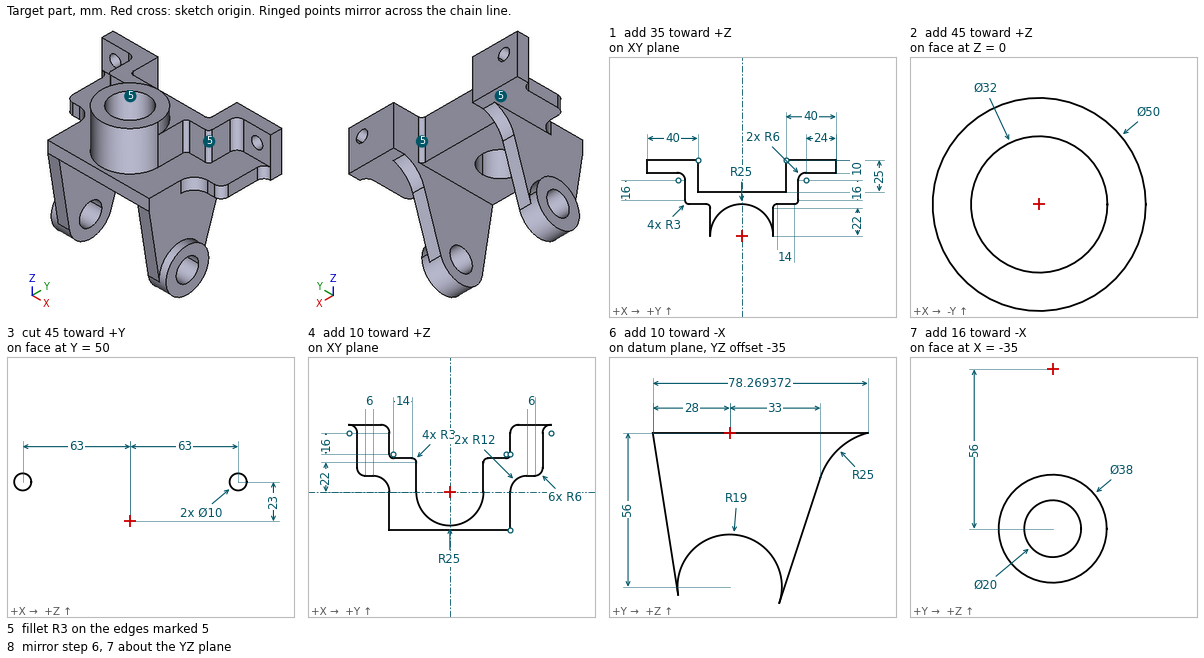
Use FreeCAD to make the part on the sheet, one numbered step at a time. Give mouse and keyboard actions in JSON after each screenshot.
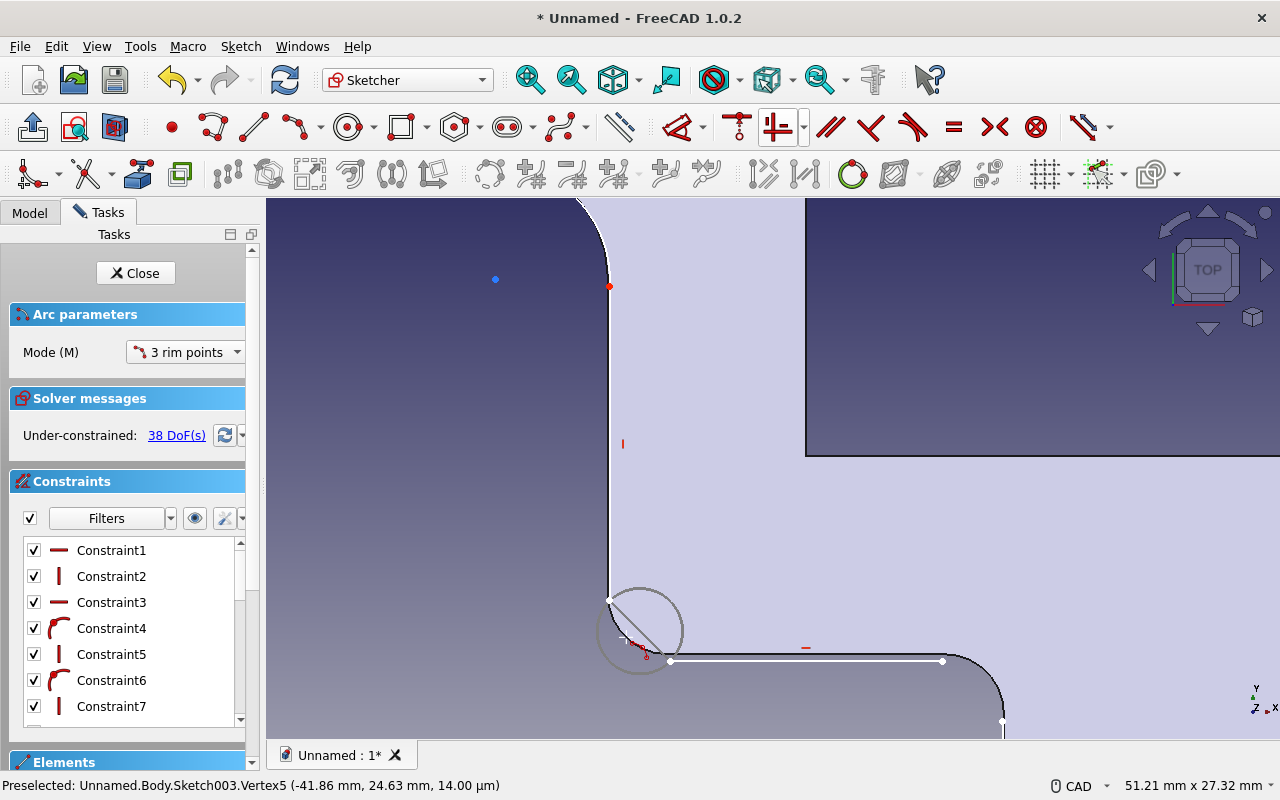
{"action": "left_click", "coordinate": [625, 637]}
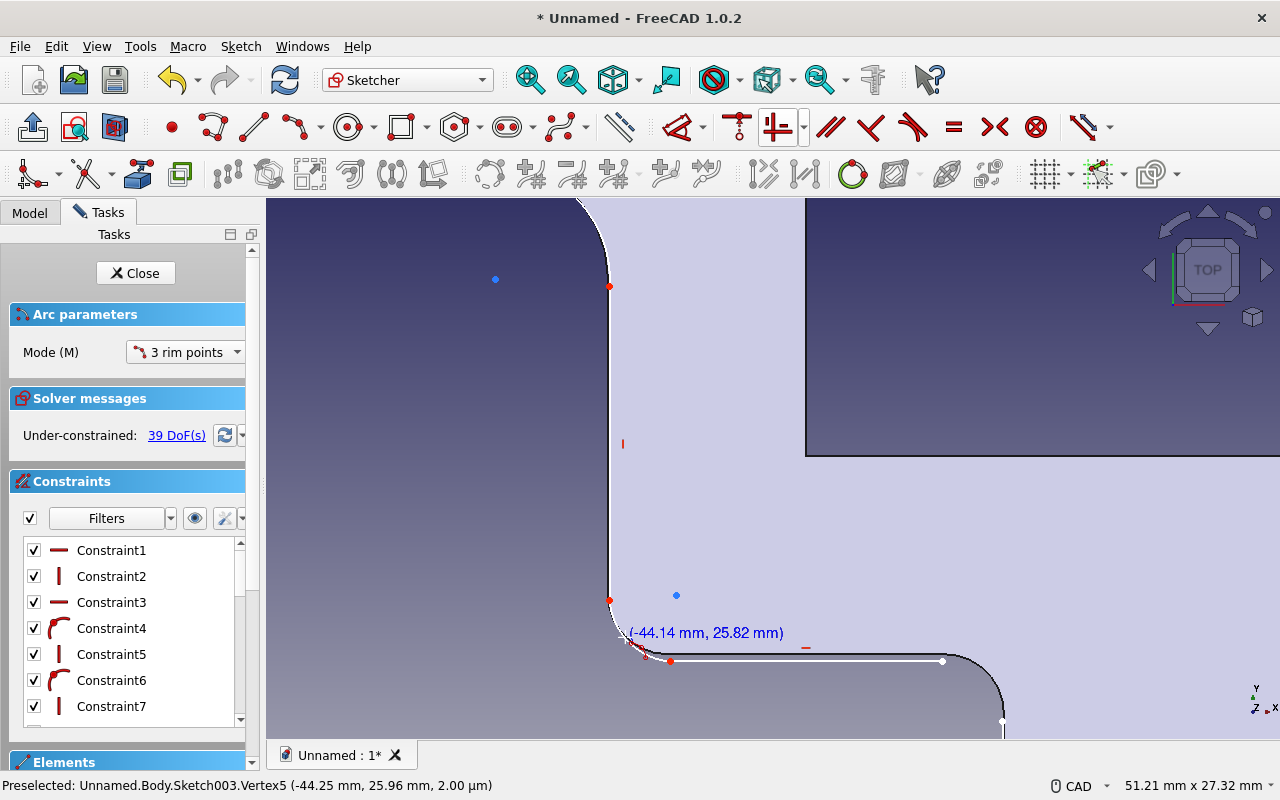
{"action": "scroll", "coordinate": [504, 351], "scroll_direction": "down", "scroll_amount": 8}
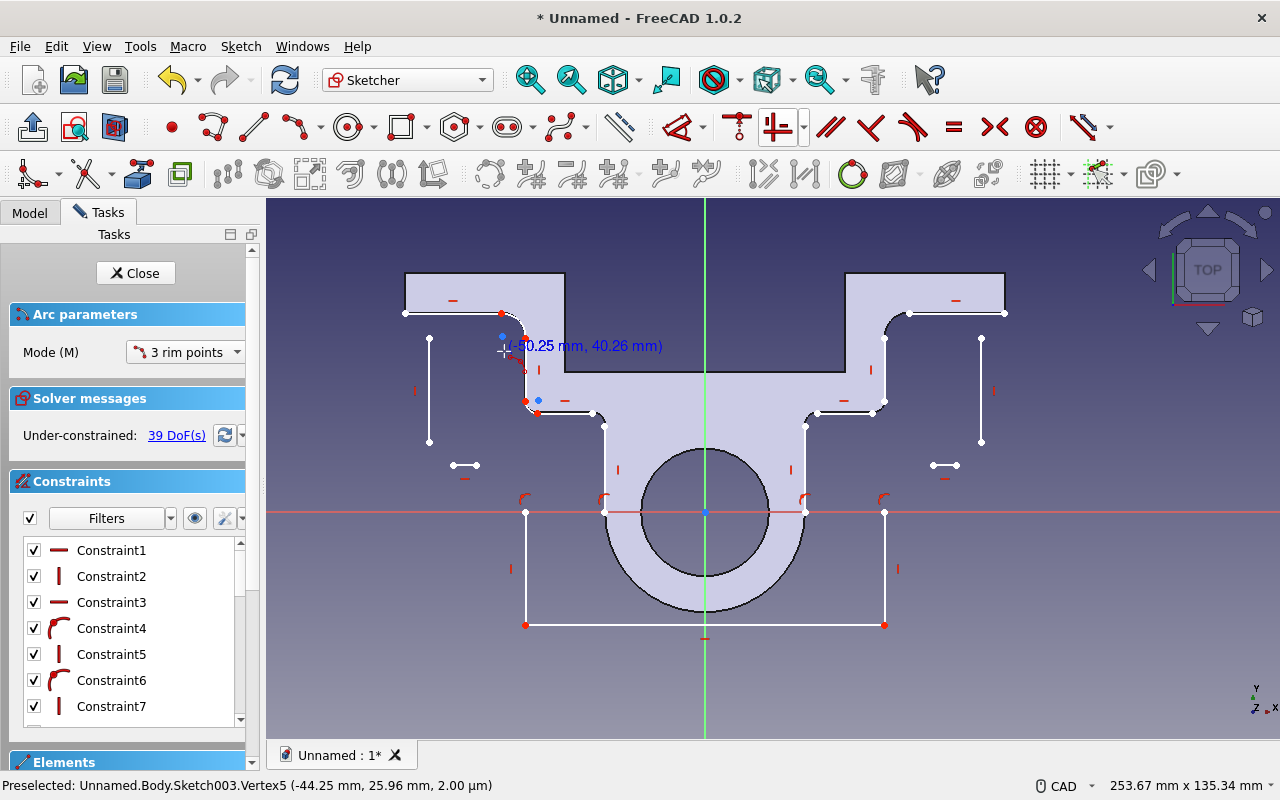
{"action": "left_click", "coordinate": [593, 414]}
{"action": "left_click", "coordinate": [605, 426]}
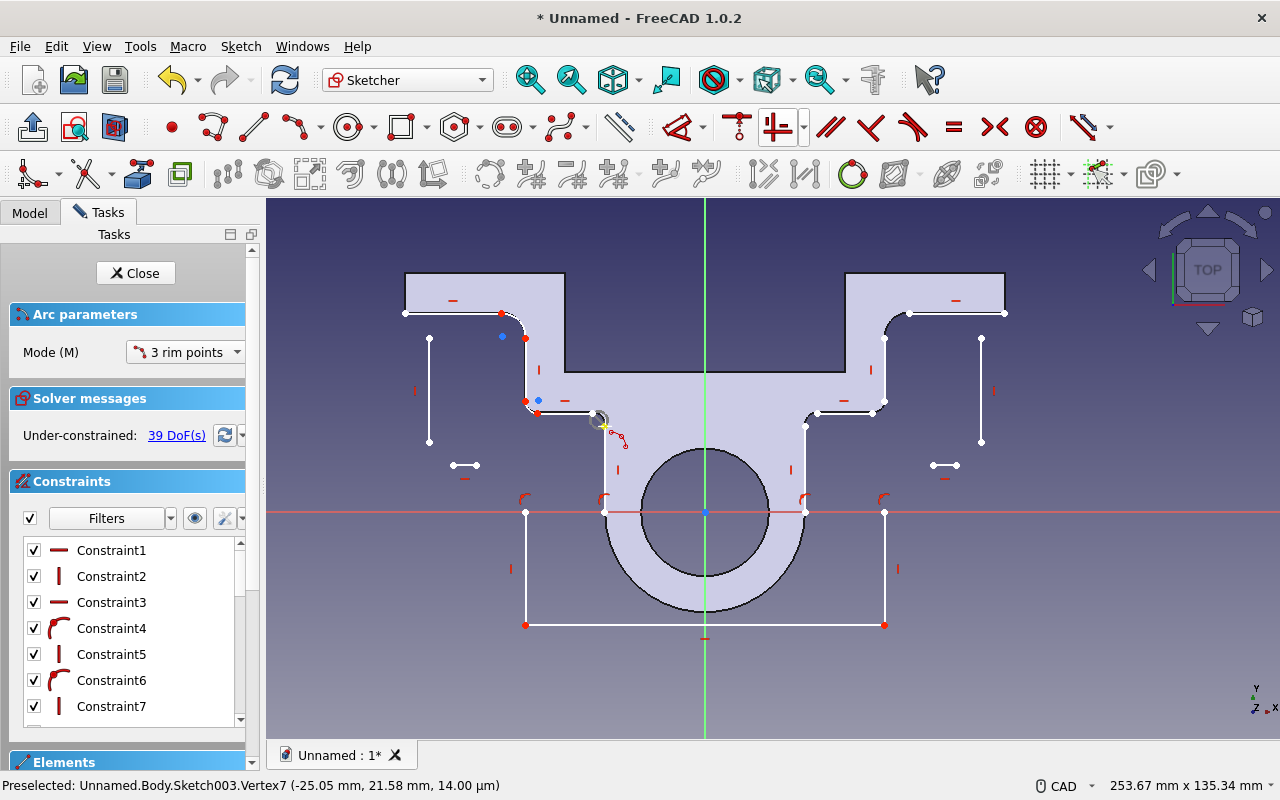
{"action": "scroll", "coordinate": [602, 416], "scroll_direction": "up", "scroll_amount": 8}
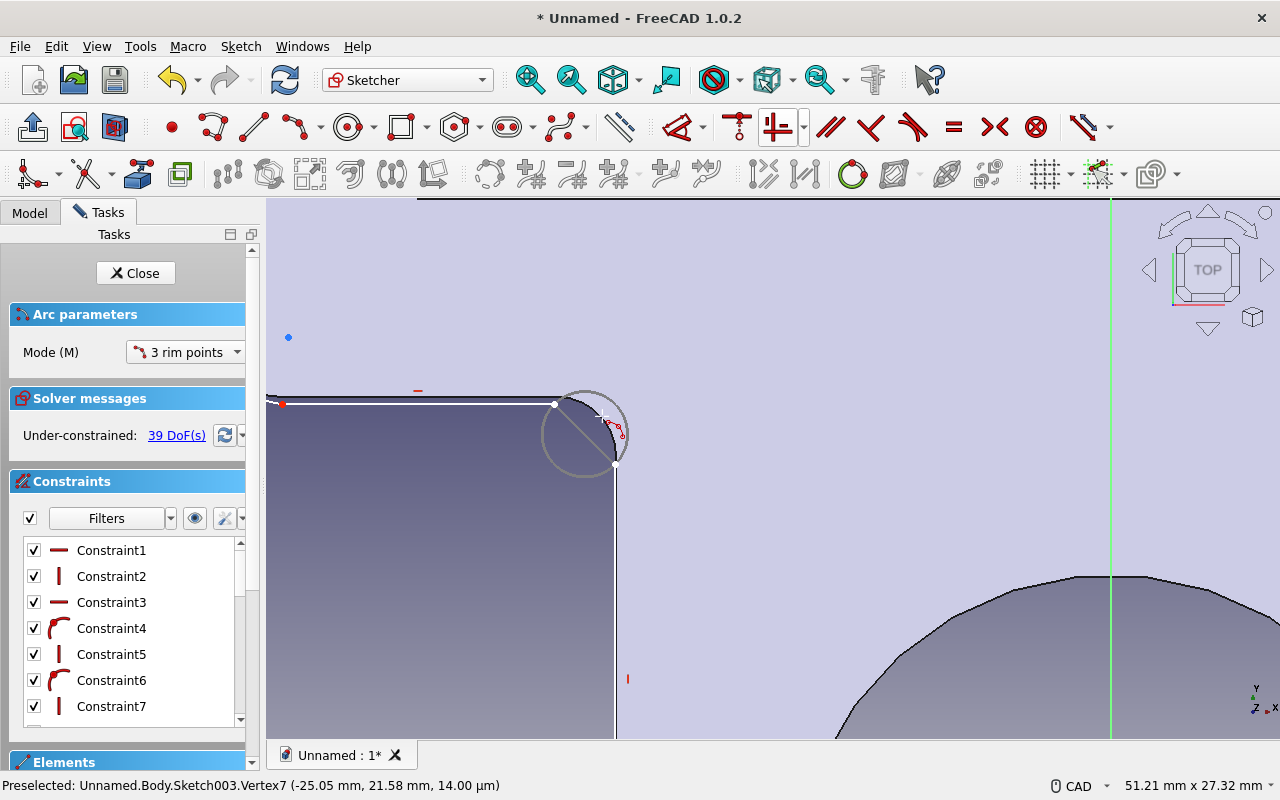
{"action": "left_click", "coordinate": [599, 414]}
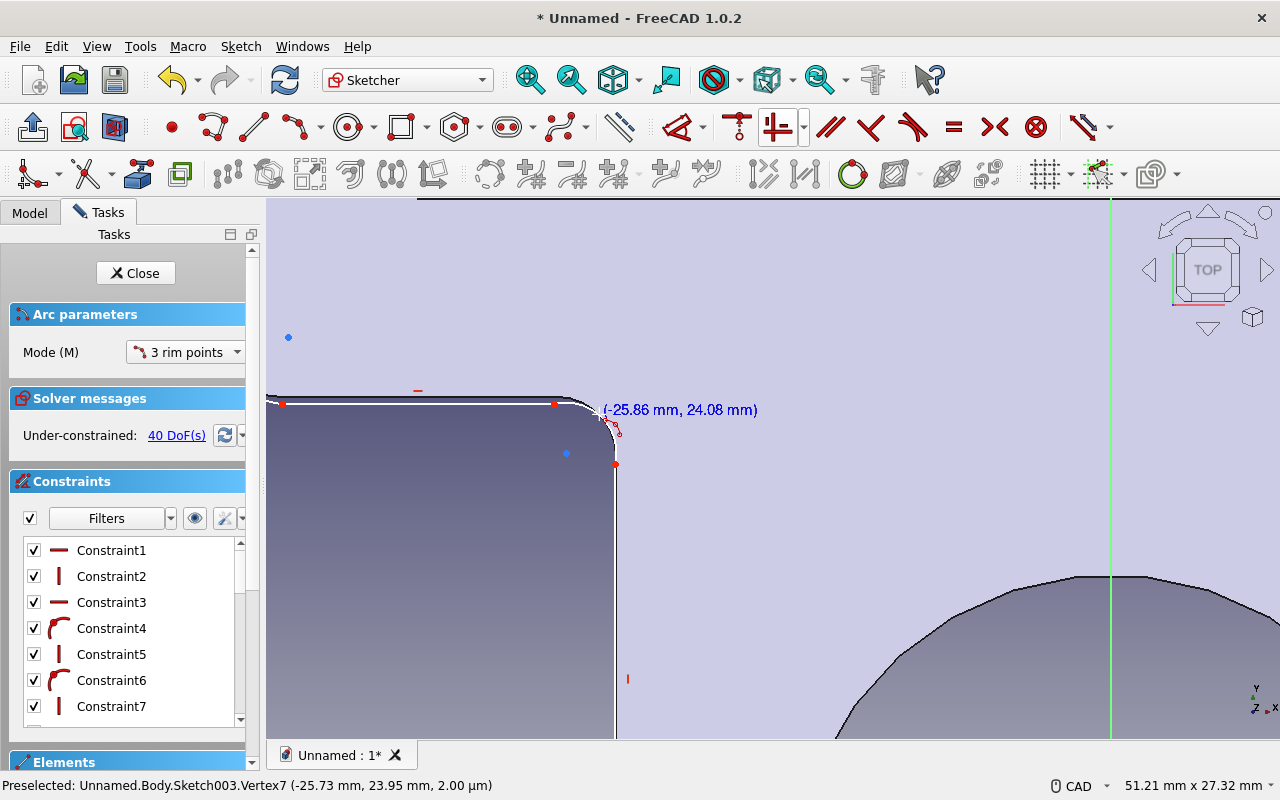
{"action": "scroll", "coordinate": [602, 417], "scroll_direction": "down", "scroll_amount": 8}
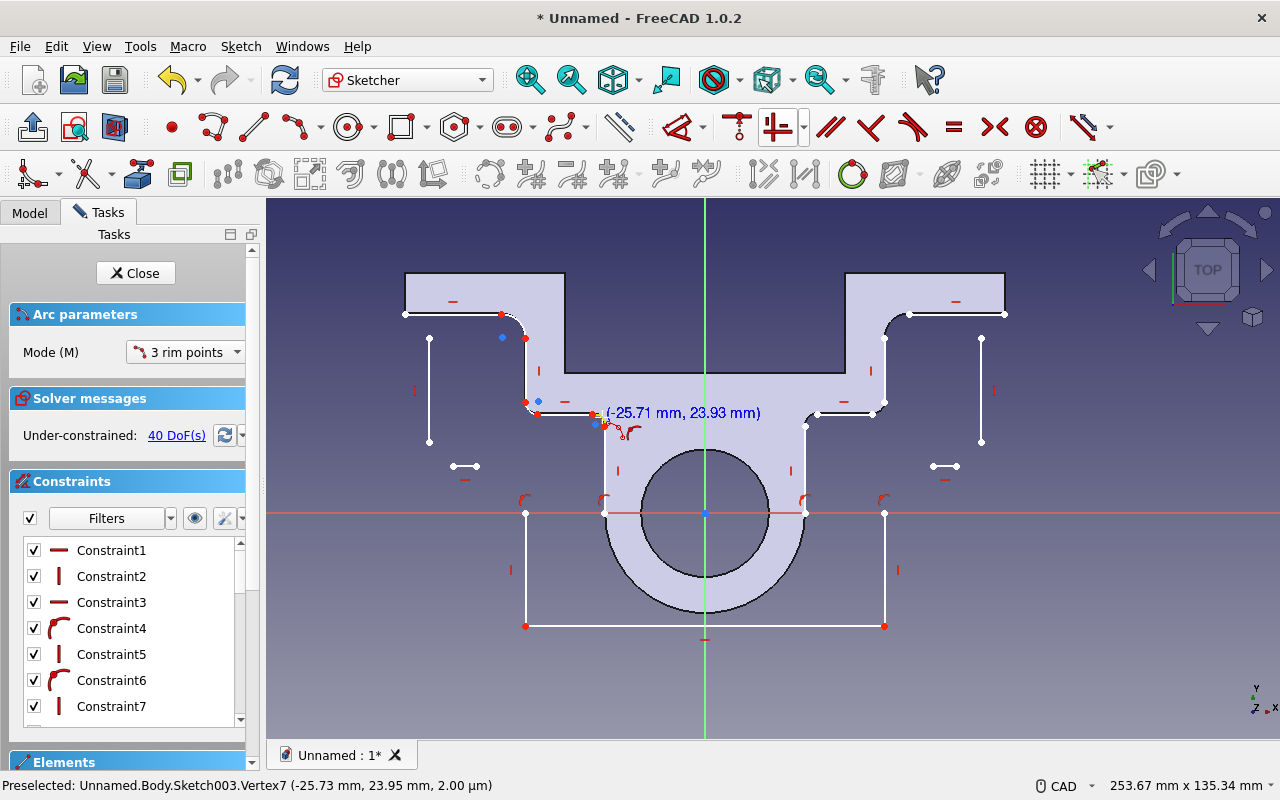
{"action": "left_click", "coordinate": [605, 513]}
{"action": "left_click", "coordinate": [805, 513]}
{"action": "left_click", "coordinate": [646, 594]}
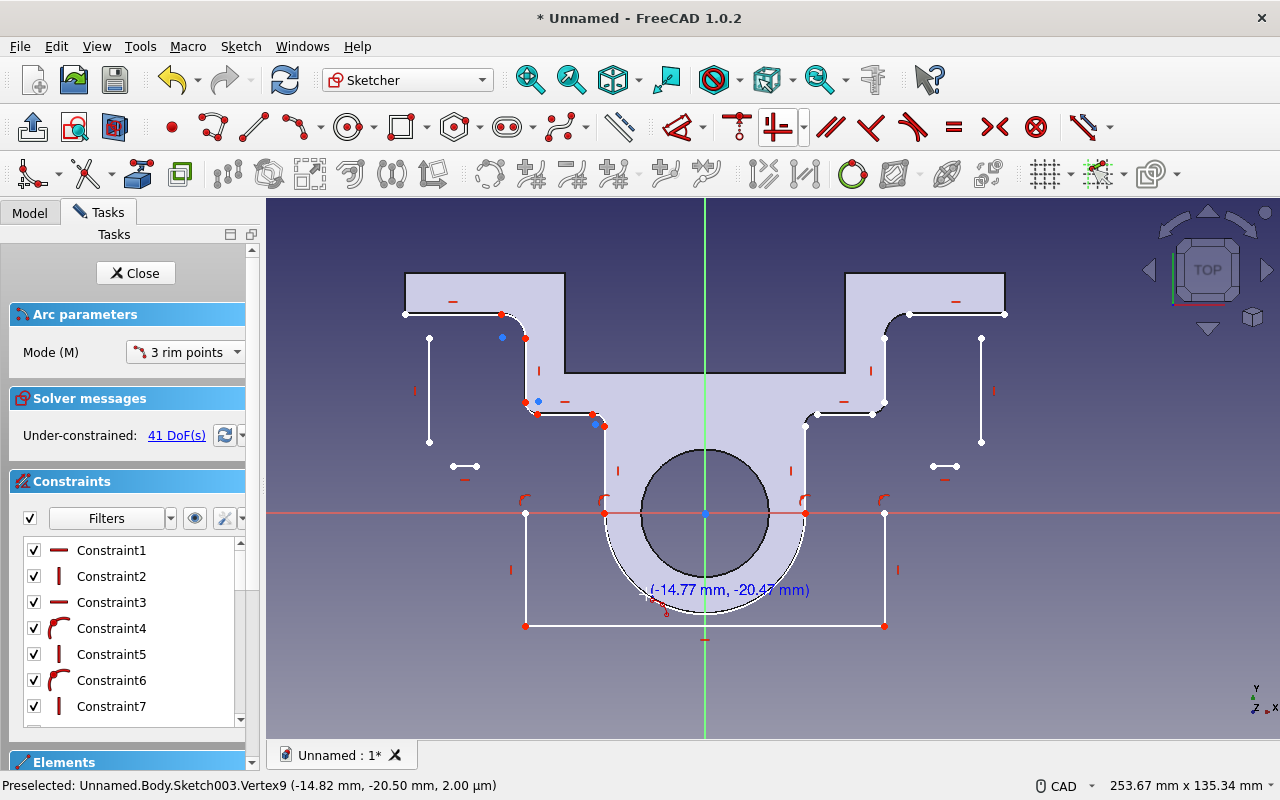
{"action": "left_click", "coordinate": [805, 427]}
{"action": "left_click", "coordinate": [817, 415]}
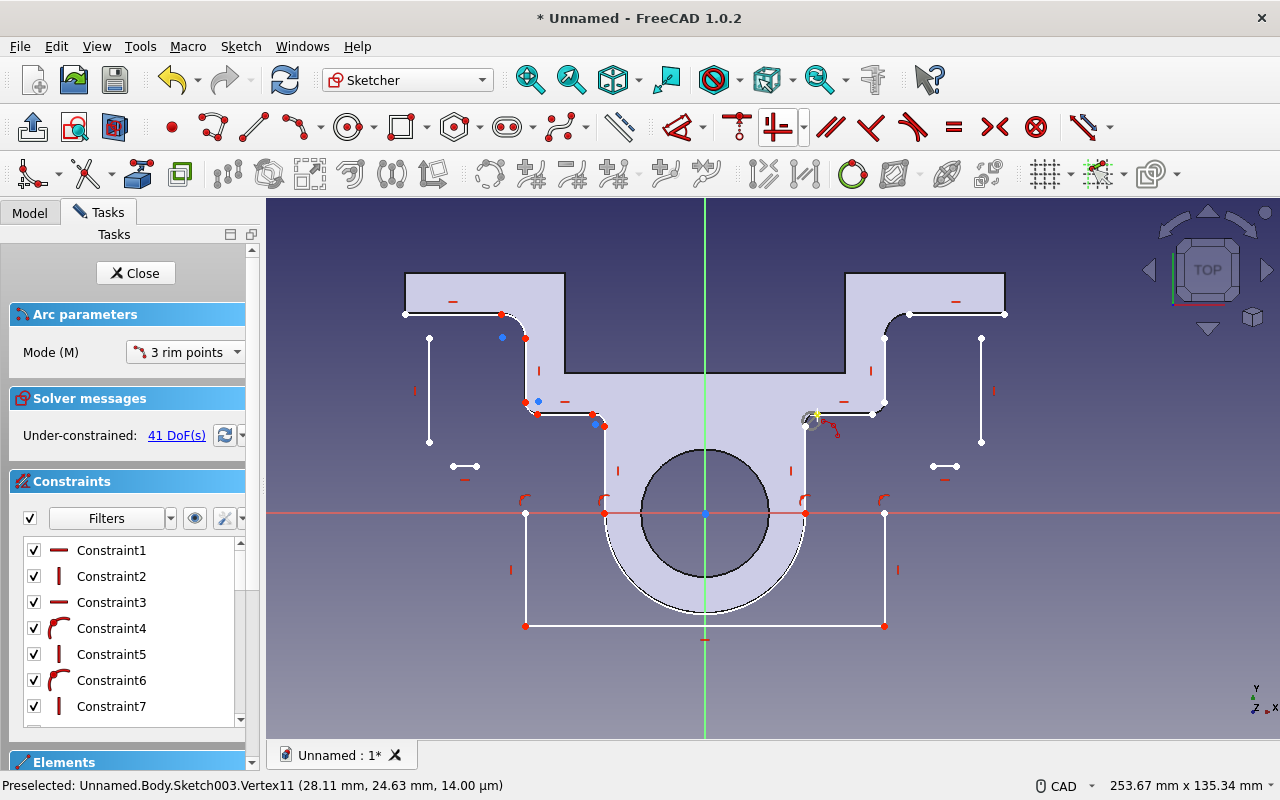
{"action": "scroll", "coordinate": [808, 417], "scroll_direction": "up", "scroll_amount": 8}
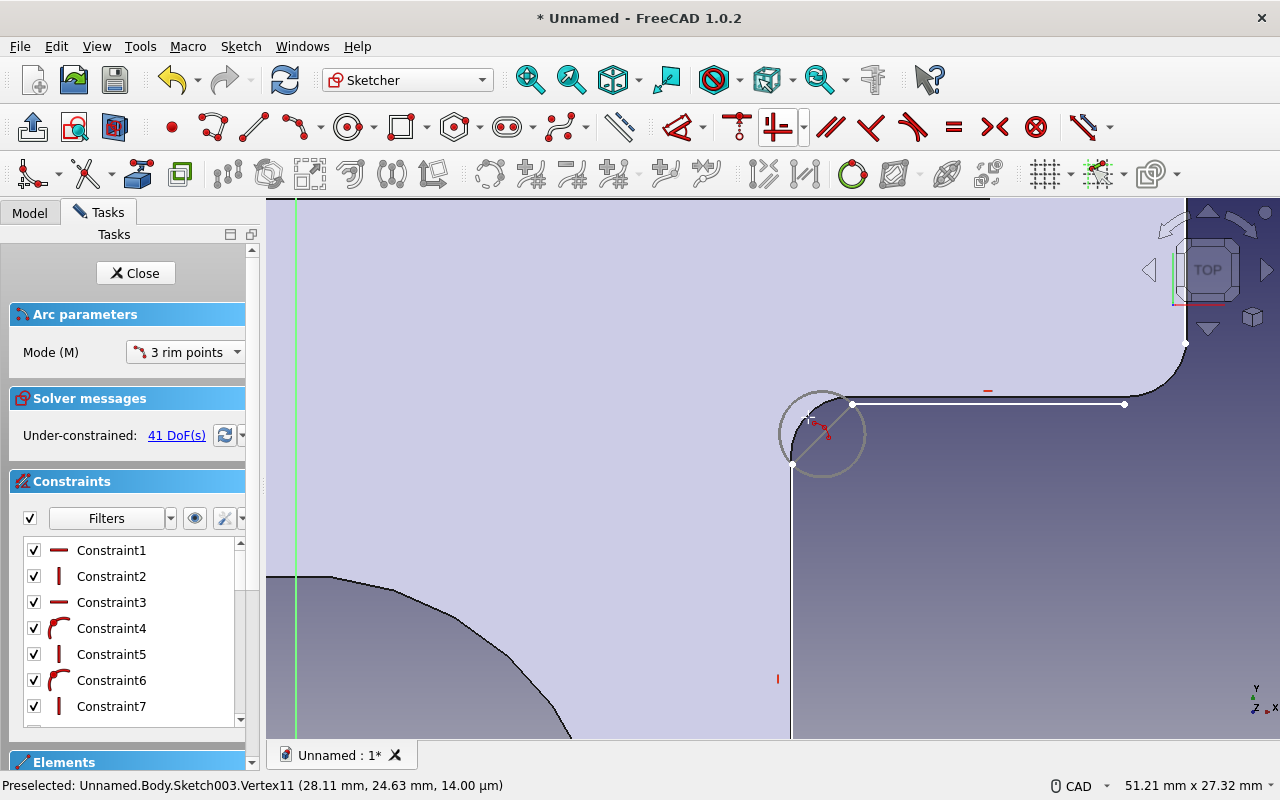
{"action": "left_click", "coordinate": [808, 414]}